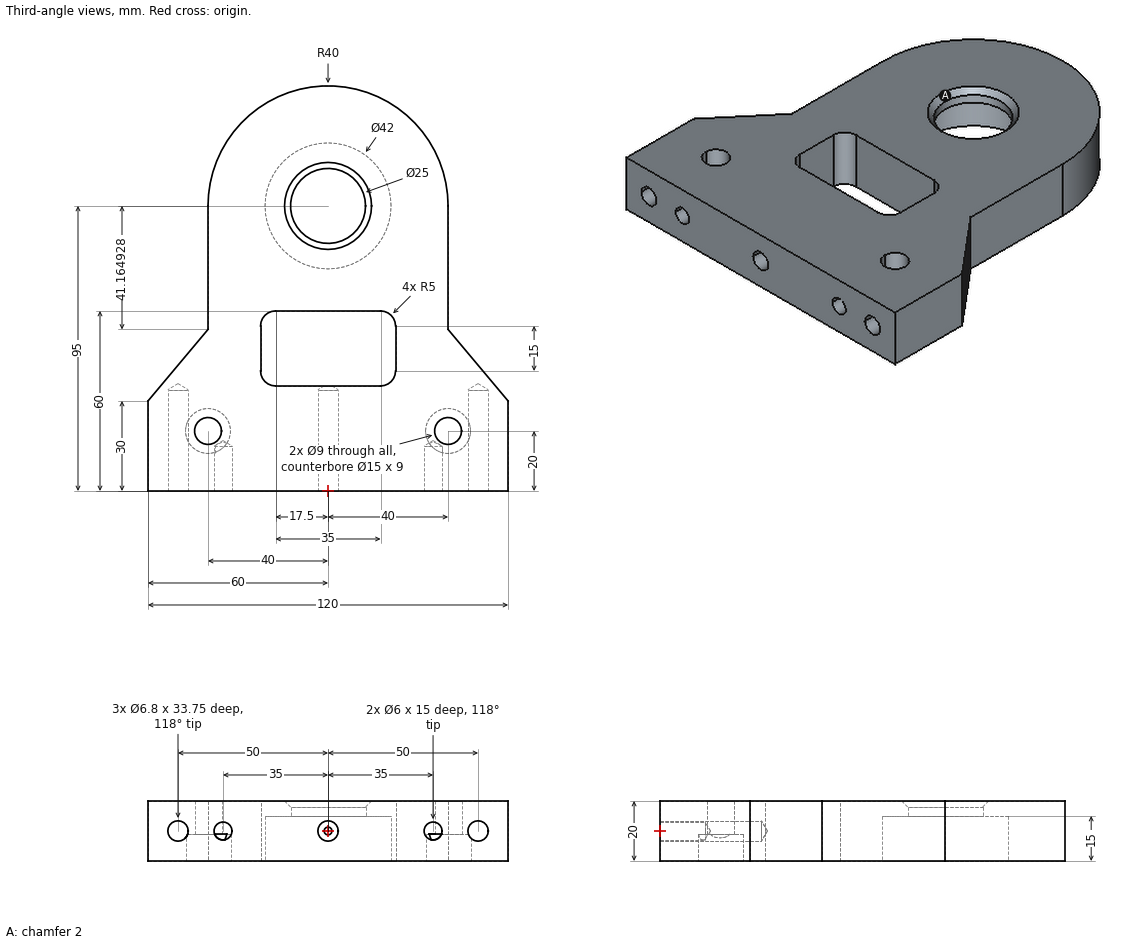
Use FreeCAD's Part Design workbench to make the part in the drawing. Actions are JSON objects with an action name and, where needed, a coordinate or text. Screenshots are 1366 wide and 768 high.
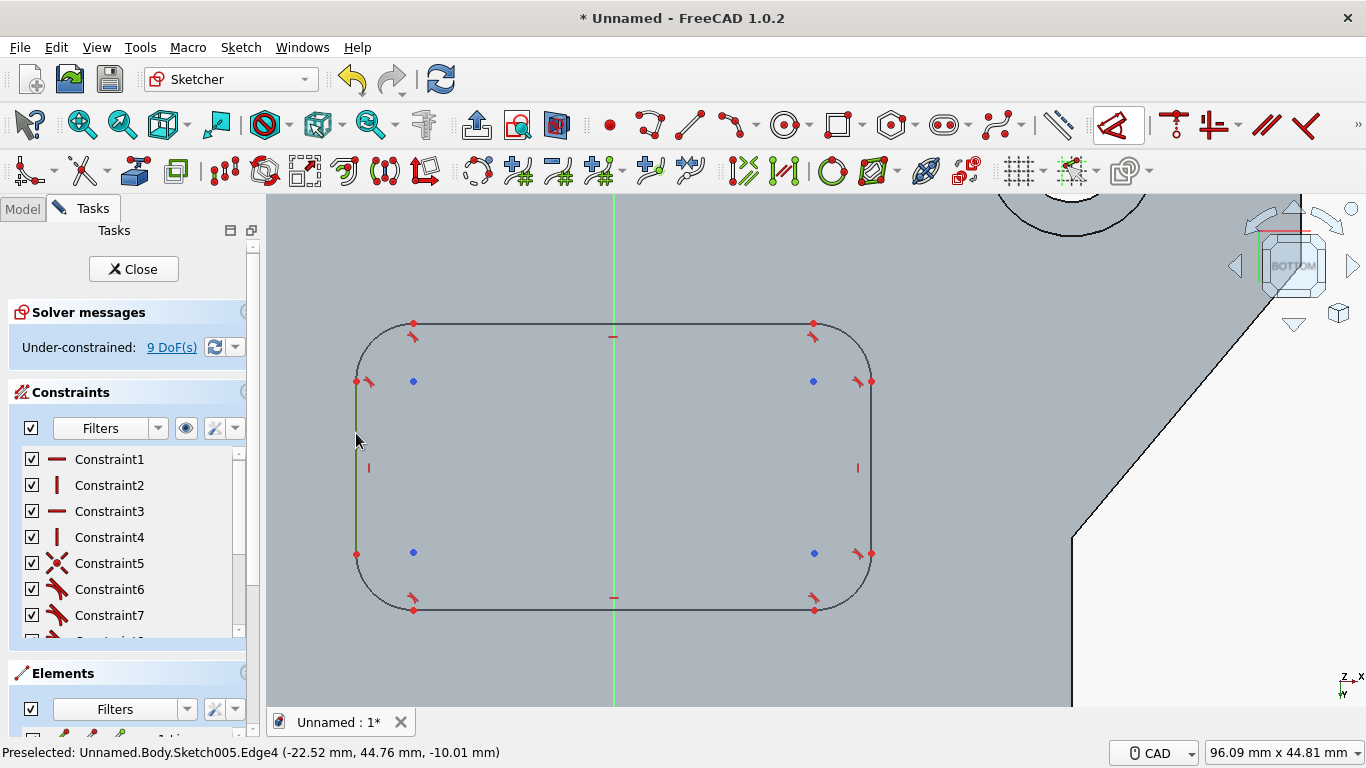
{"action": "left_click", "coordinate": [363, 580]}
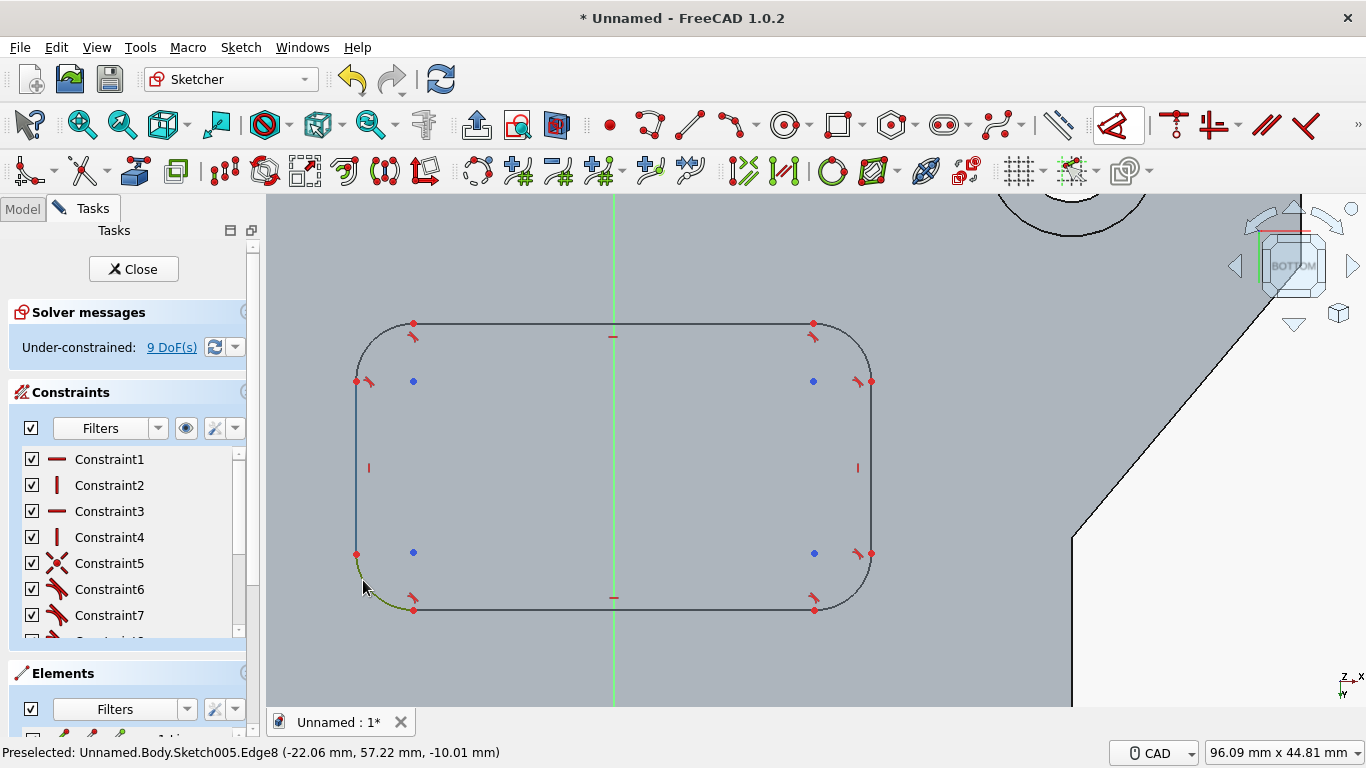
{"action": "key", "text": "t"}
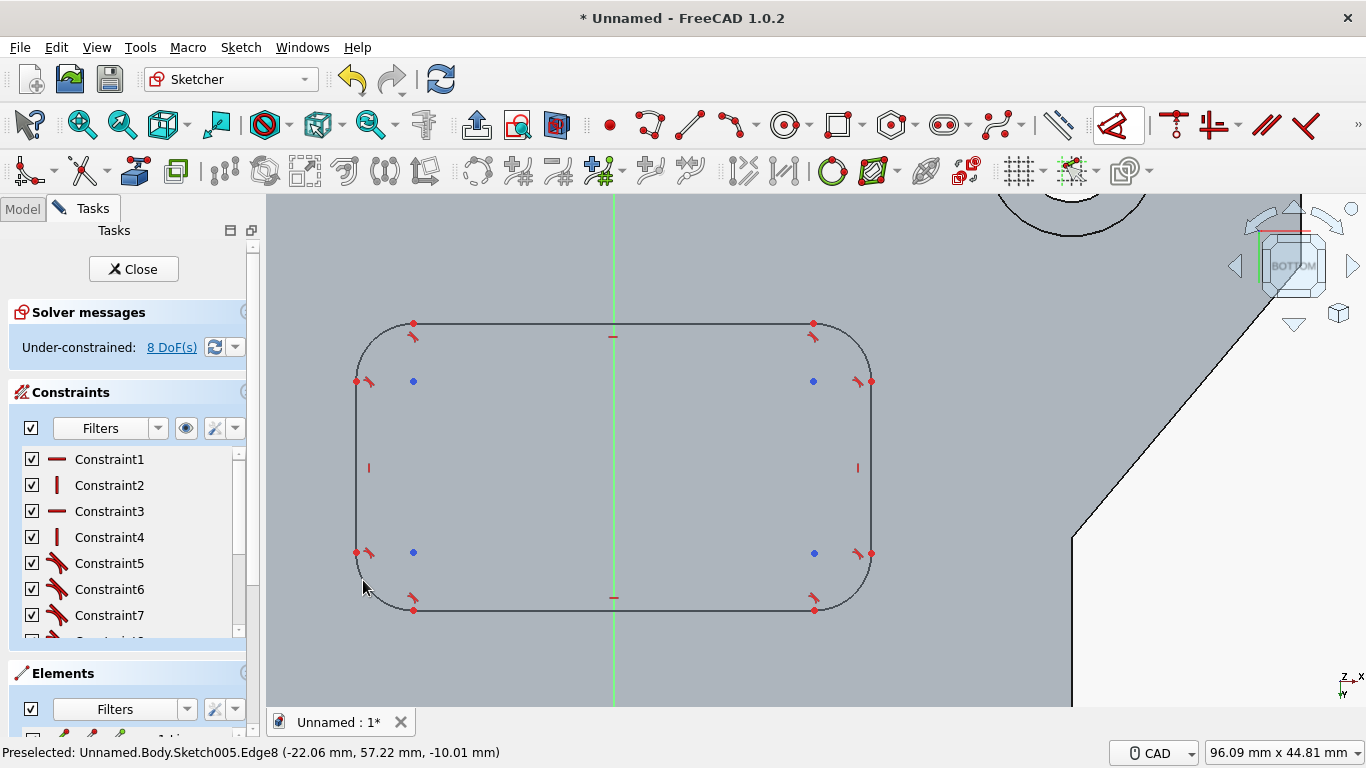
{"action": "left_click", "coordinate": [840, 604]}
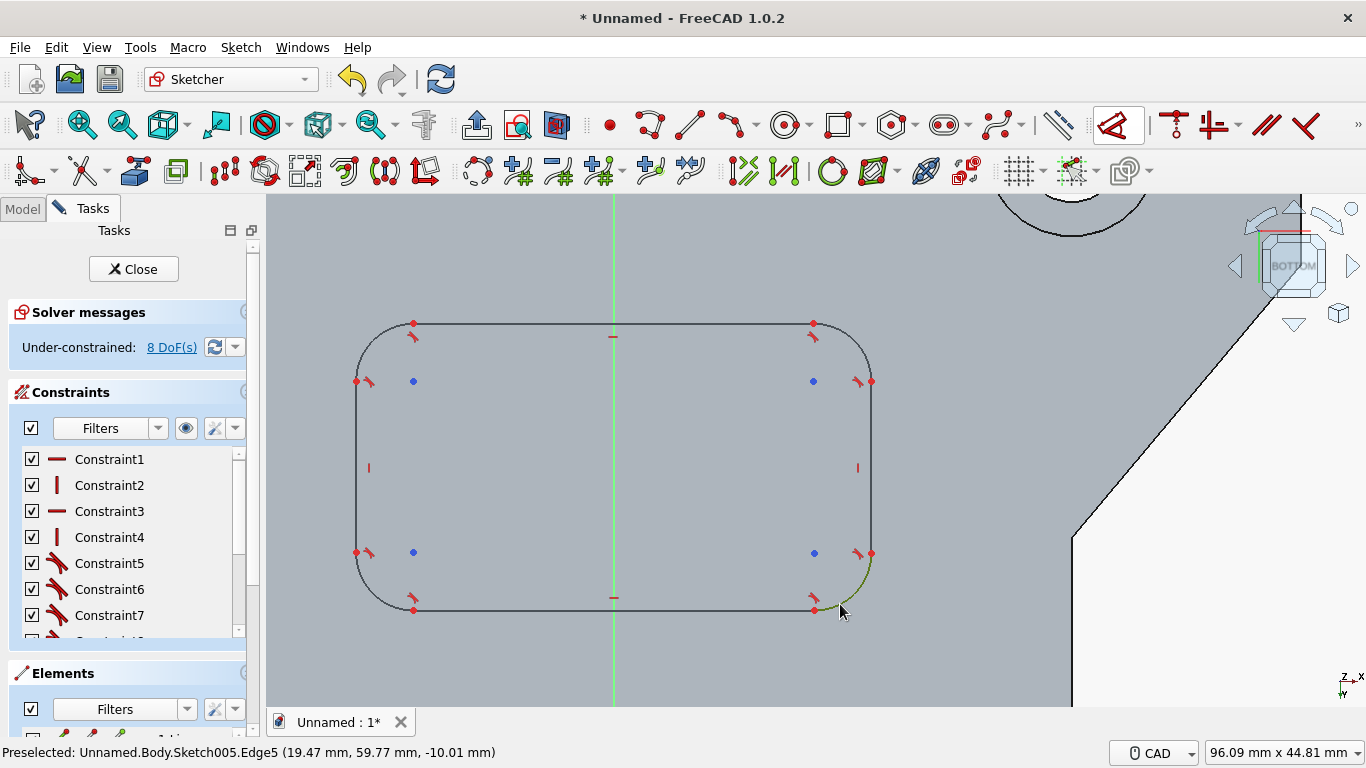
{"action": "left_click", "coordinate": [865, 355]}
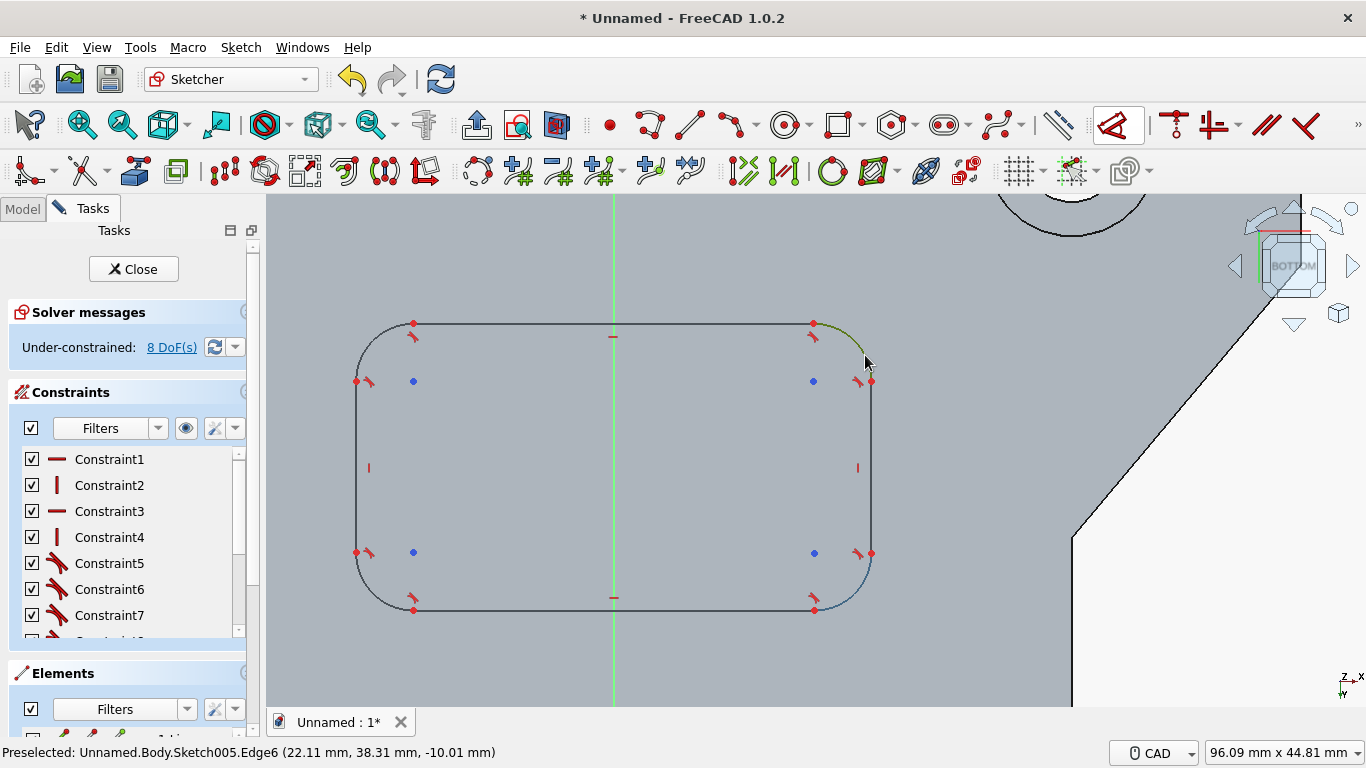
{"action": "left_click", "coordinate": [388, 330]}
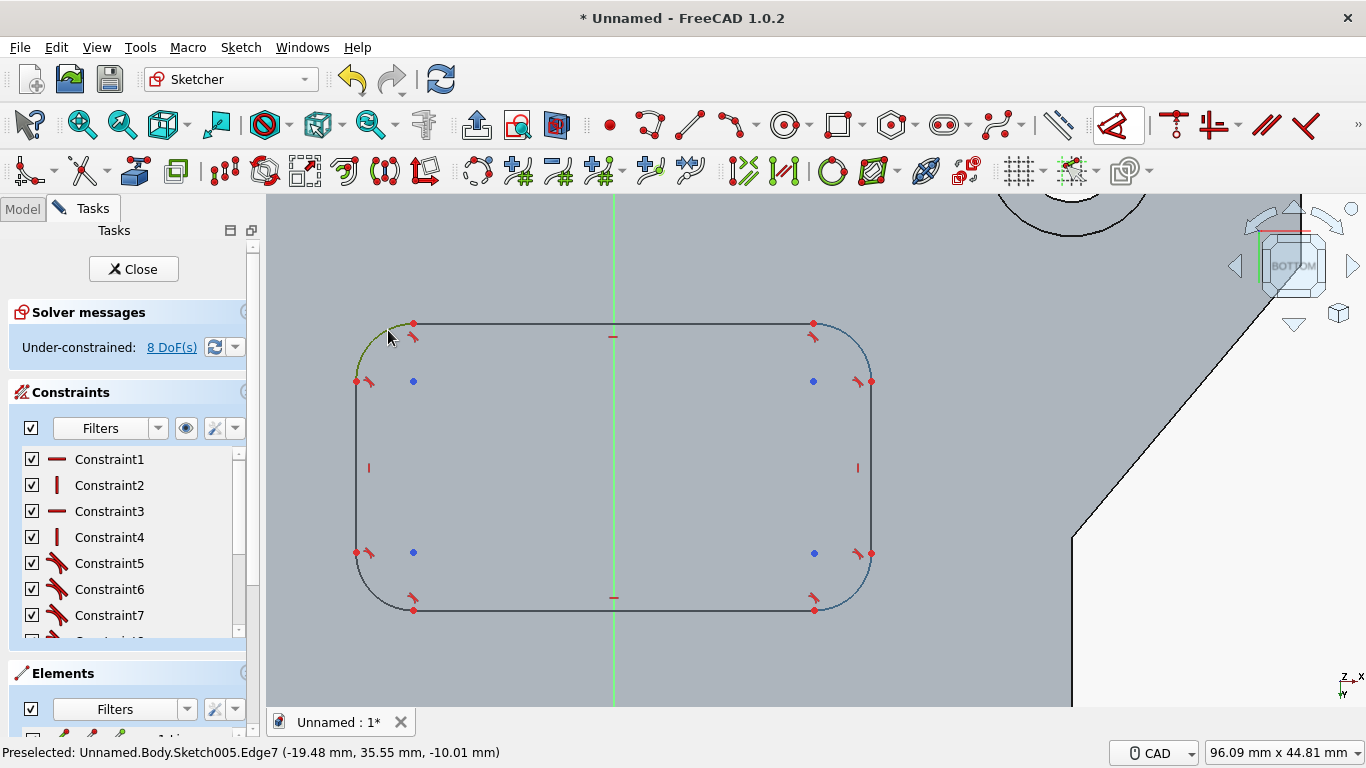
{"action": "left_click", "coordinate": [362, 579]}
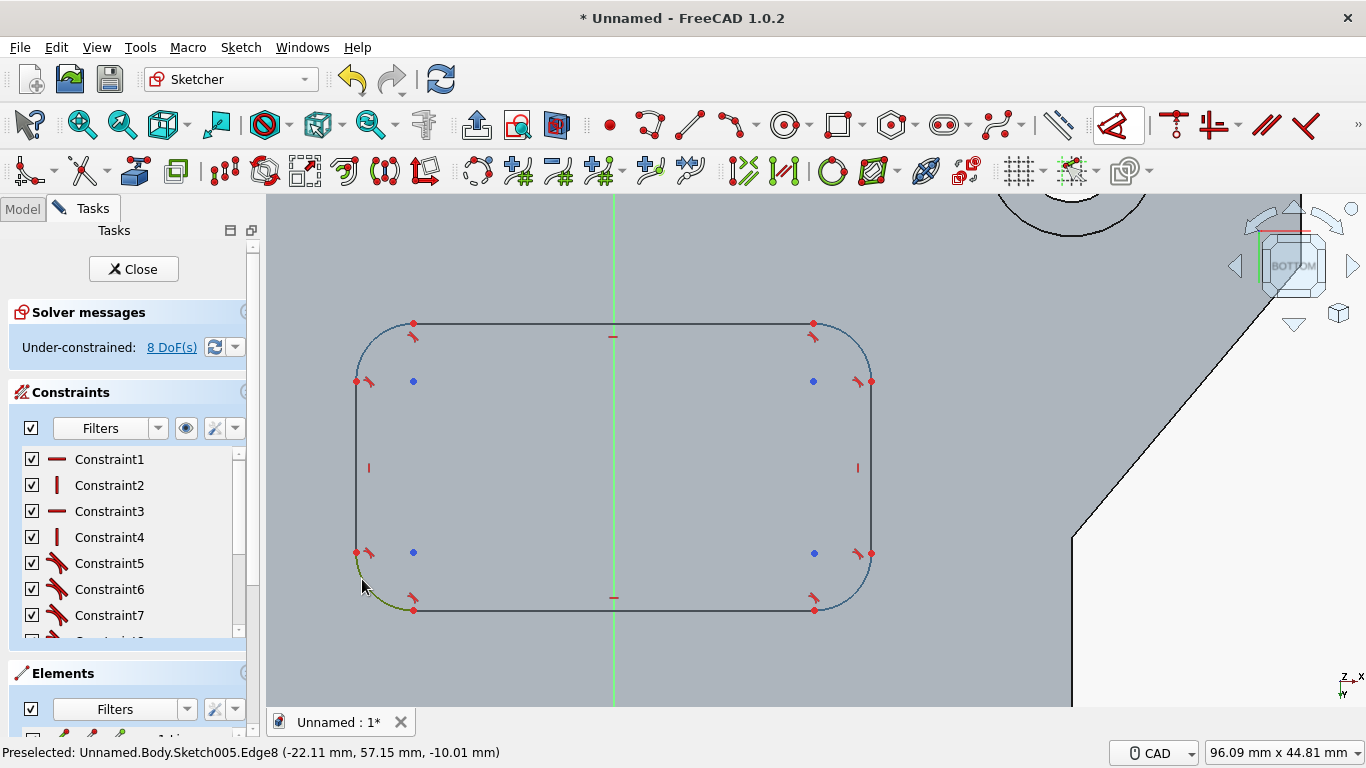
{"action": "key", "text": "e"}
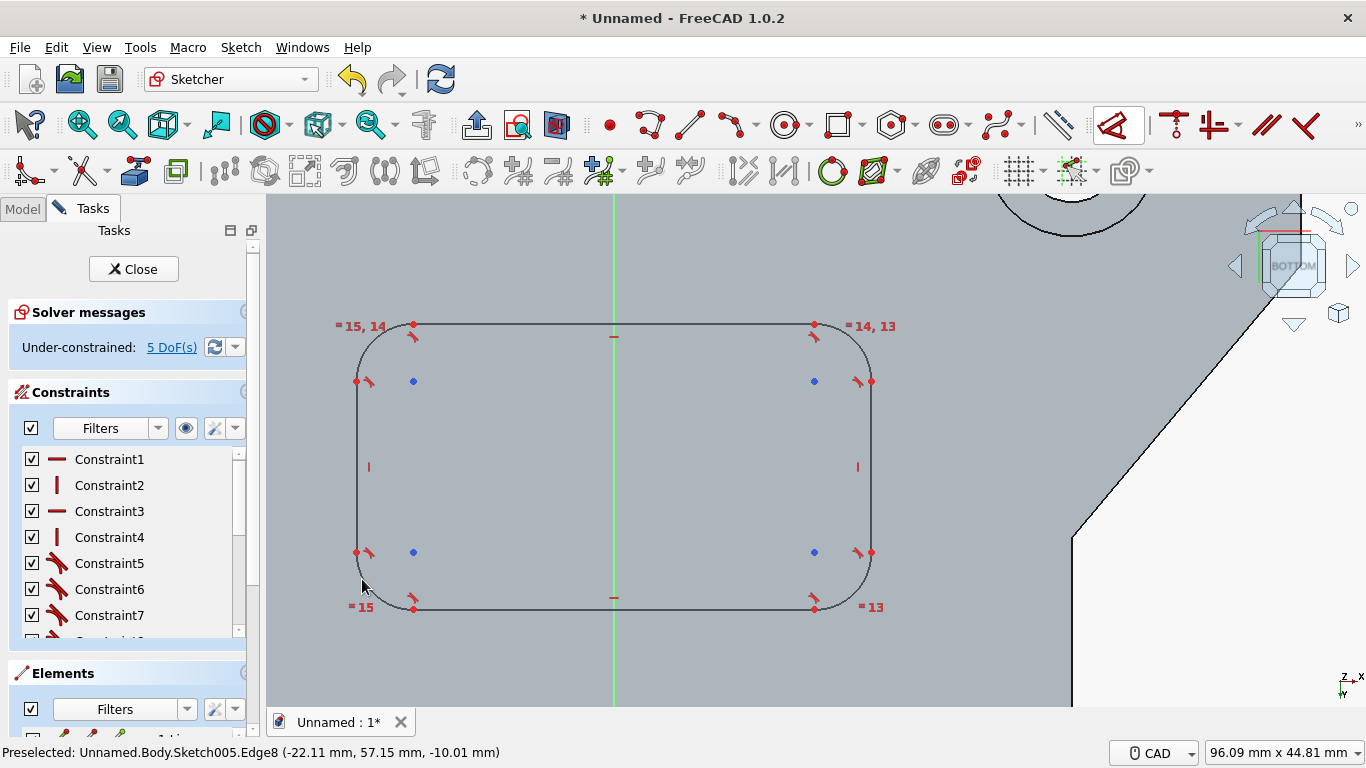
{"action": "left_click", "coordinate": [840, 604]}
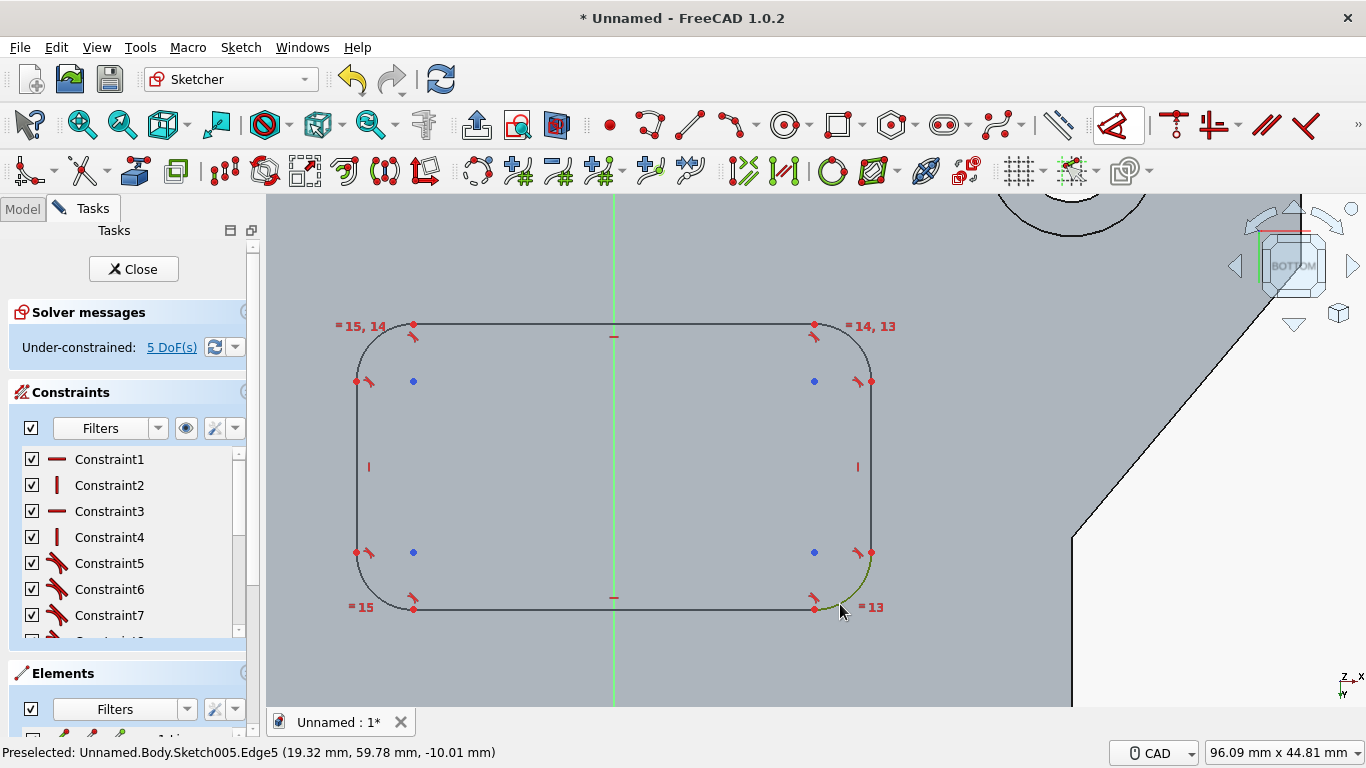
{"action": "left_click", "coordinate": [1138, 126]}